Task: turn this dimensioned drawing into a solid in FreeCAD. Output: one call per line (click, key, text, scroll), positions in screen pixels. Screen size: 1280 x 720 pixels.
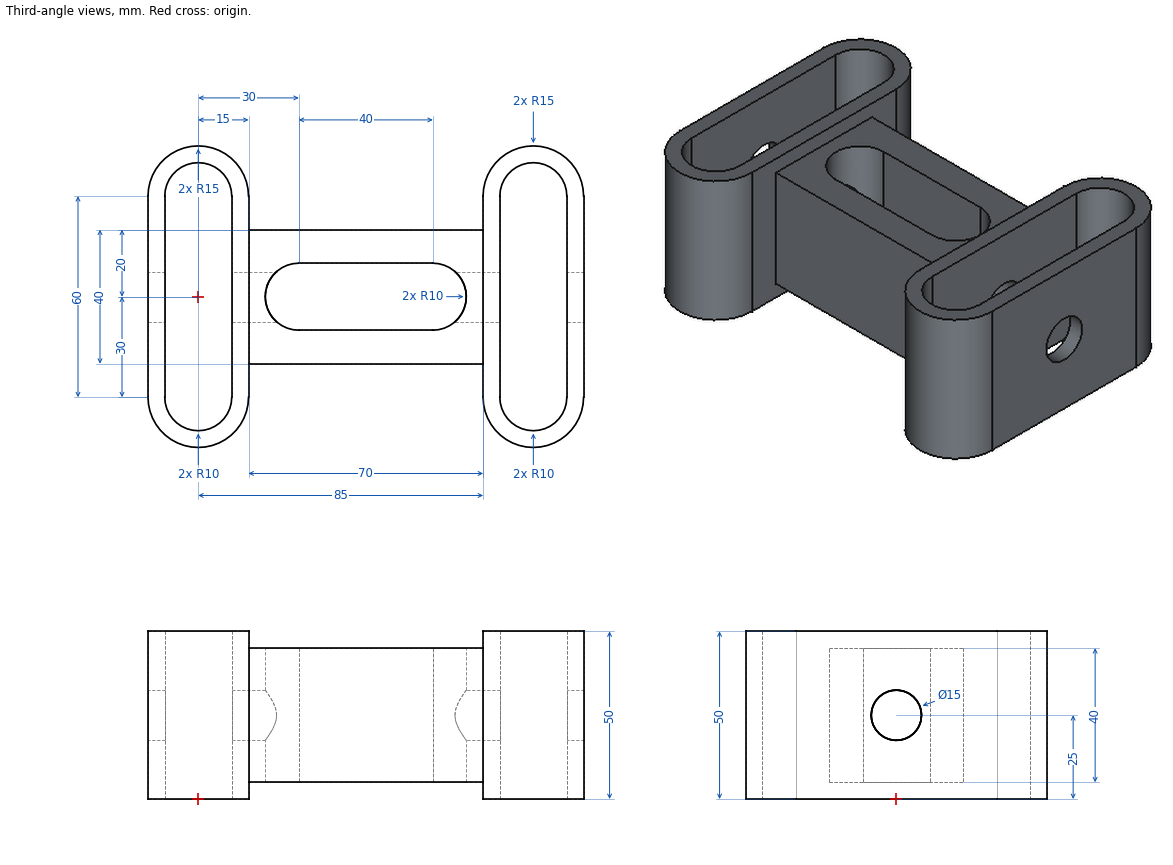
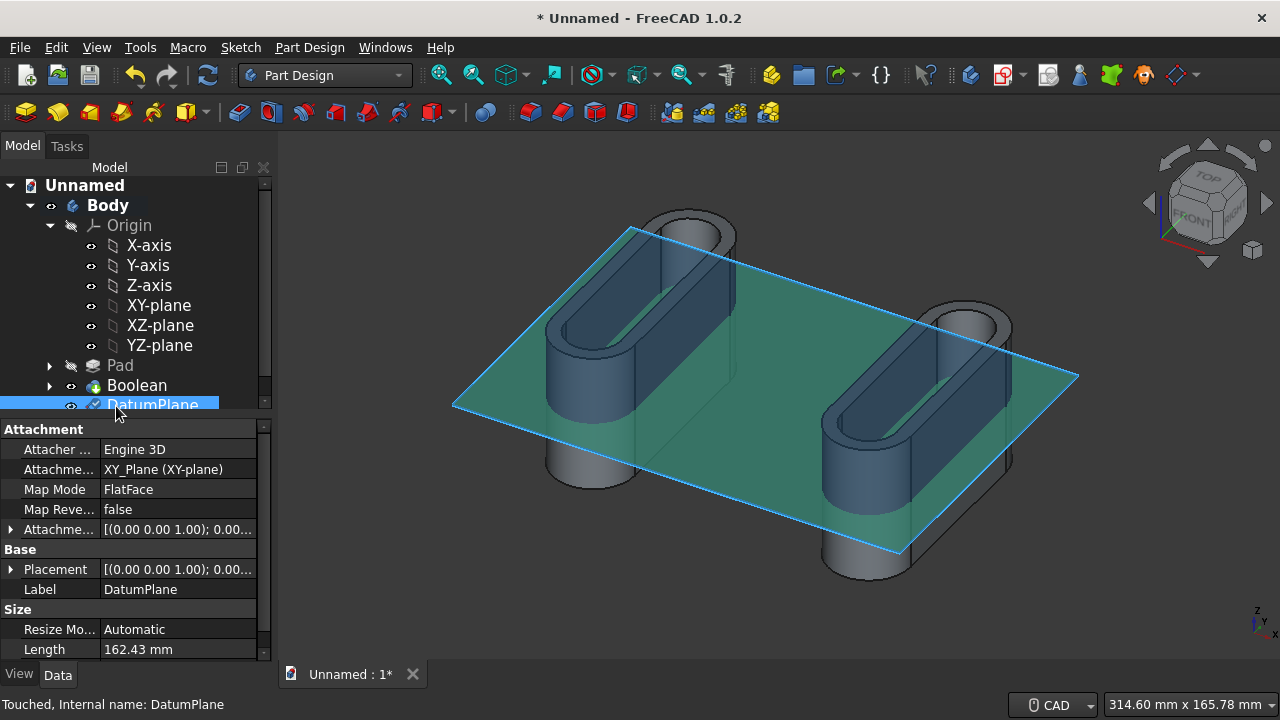
click(1004, 76)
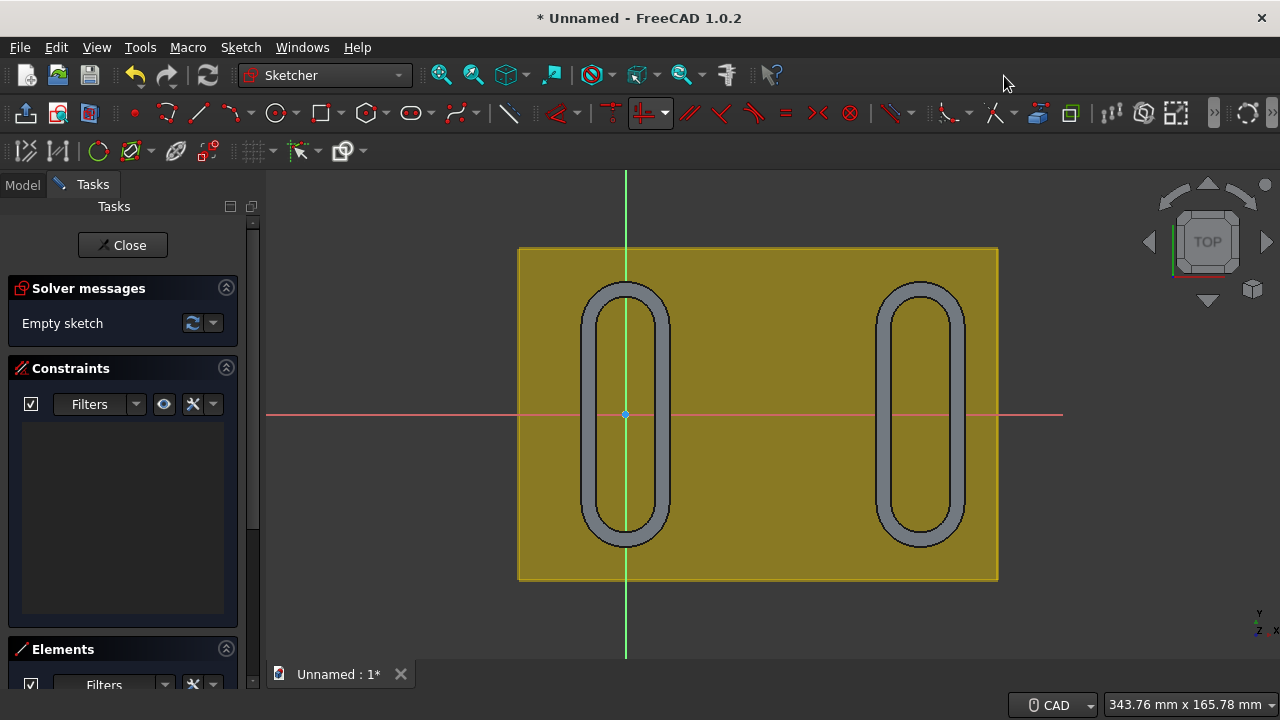
click(90, 114)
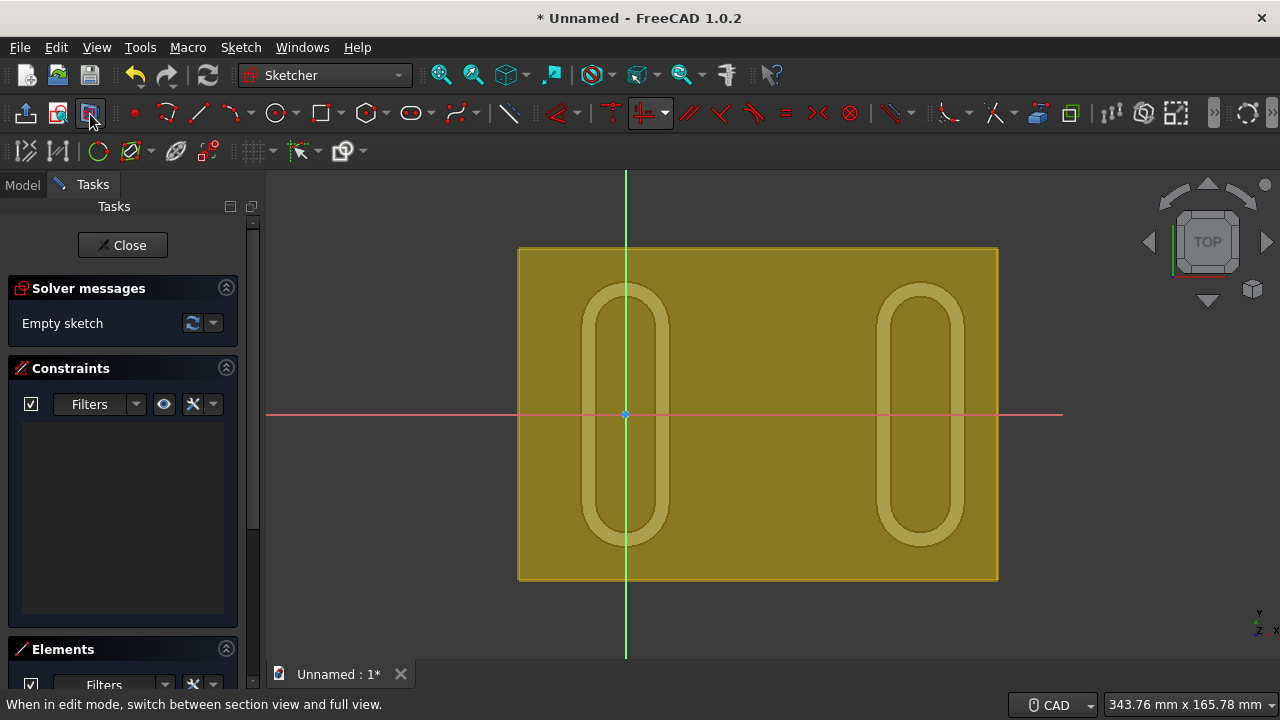
scroll(789, 414, up, 4)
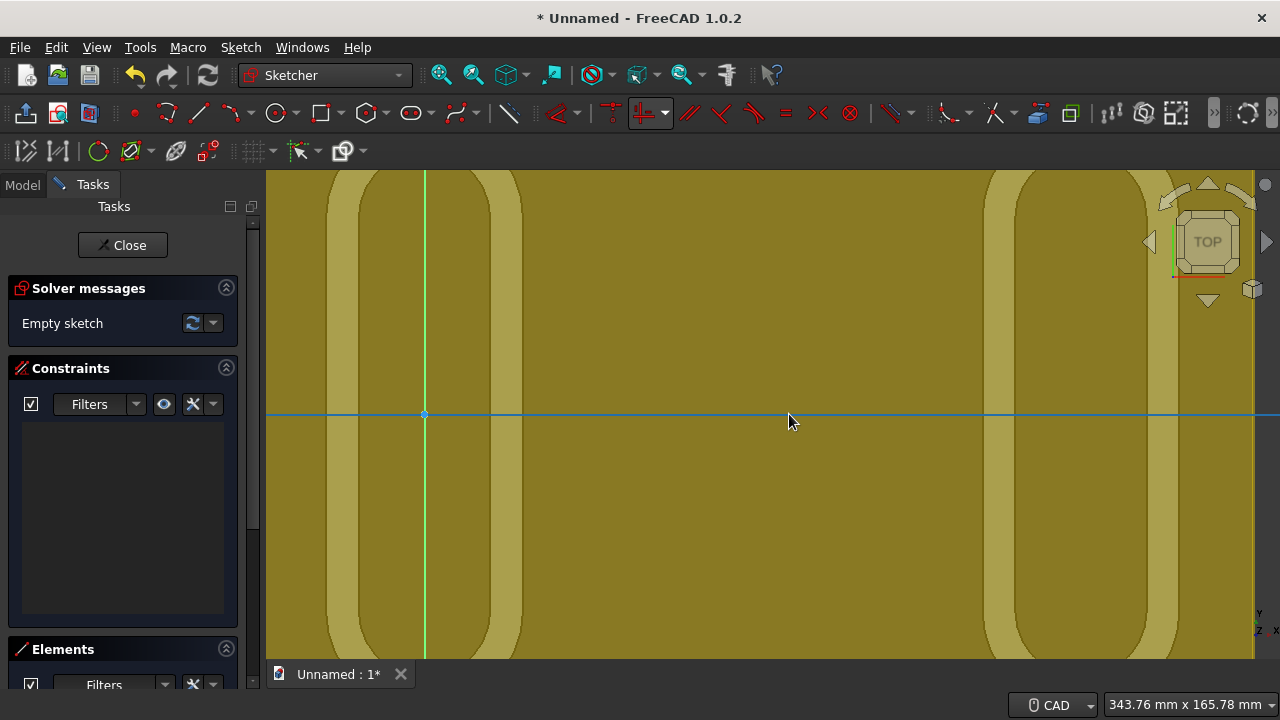
click(322, 114)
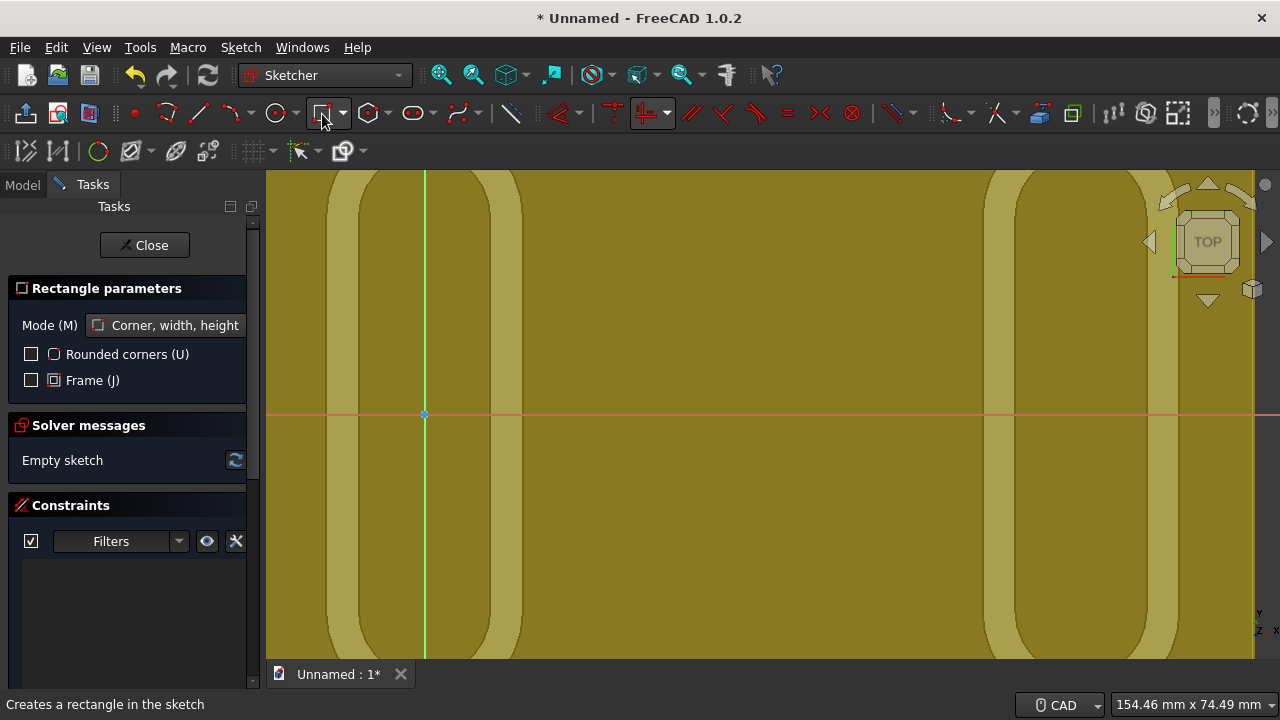
click(523, 283)
click(983, 546)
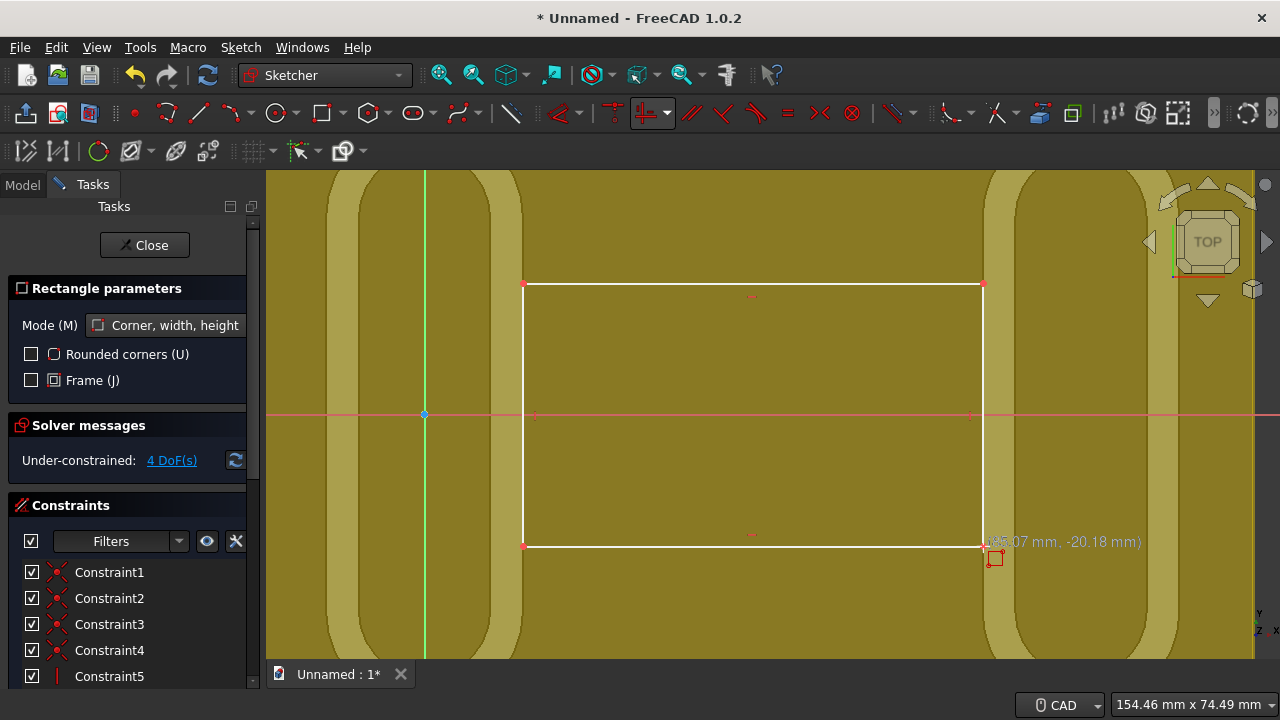
click(414, 114)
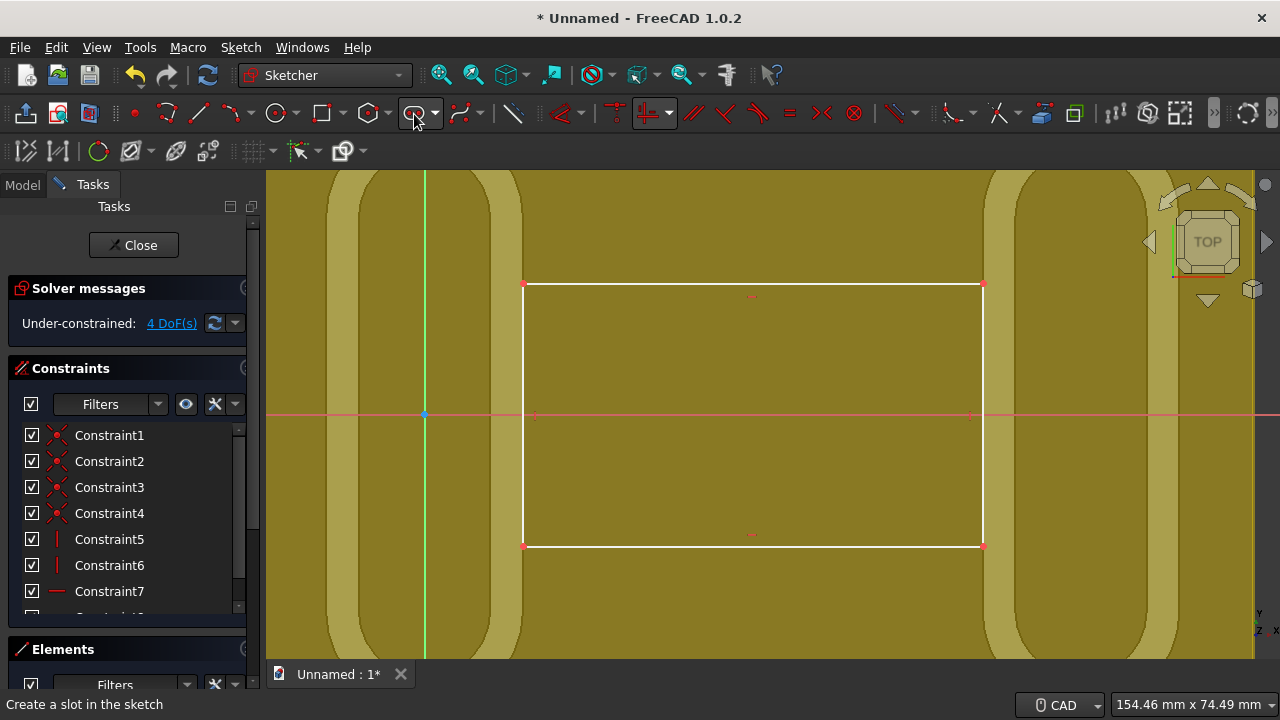
click(621, 414)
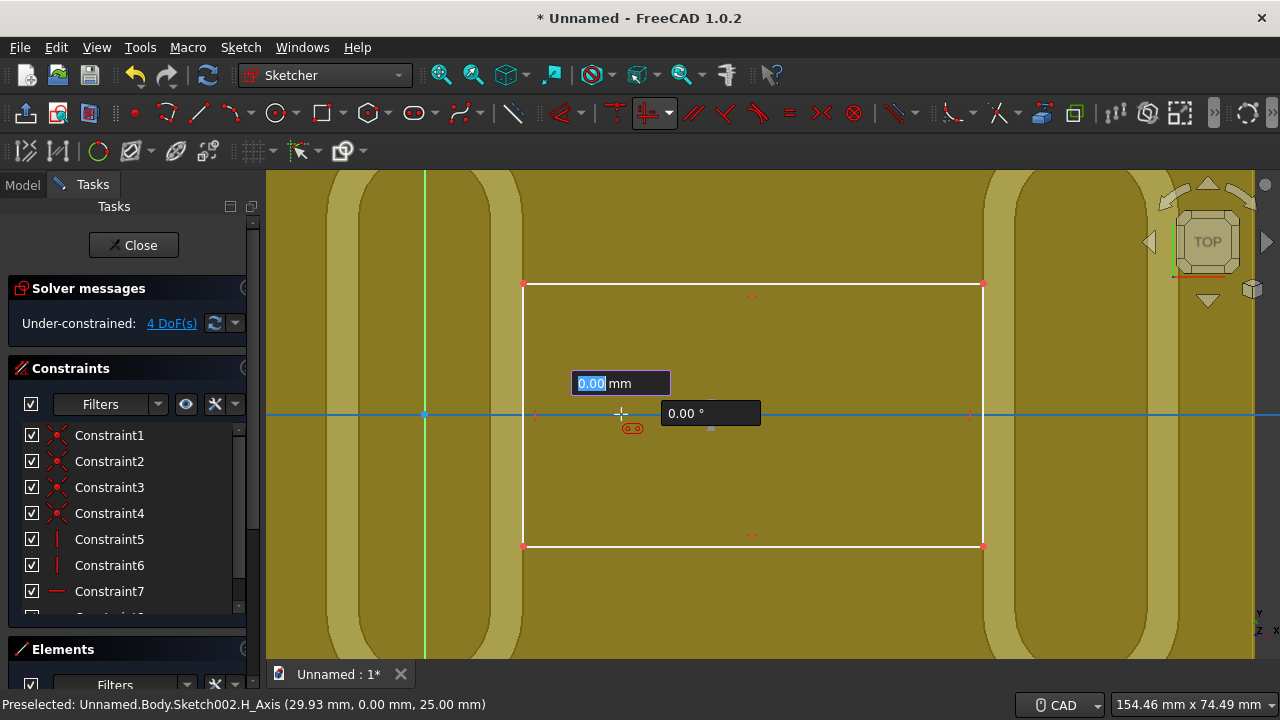
click(884, 406)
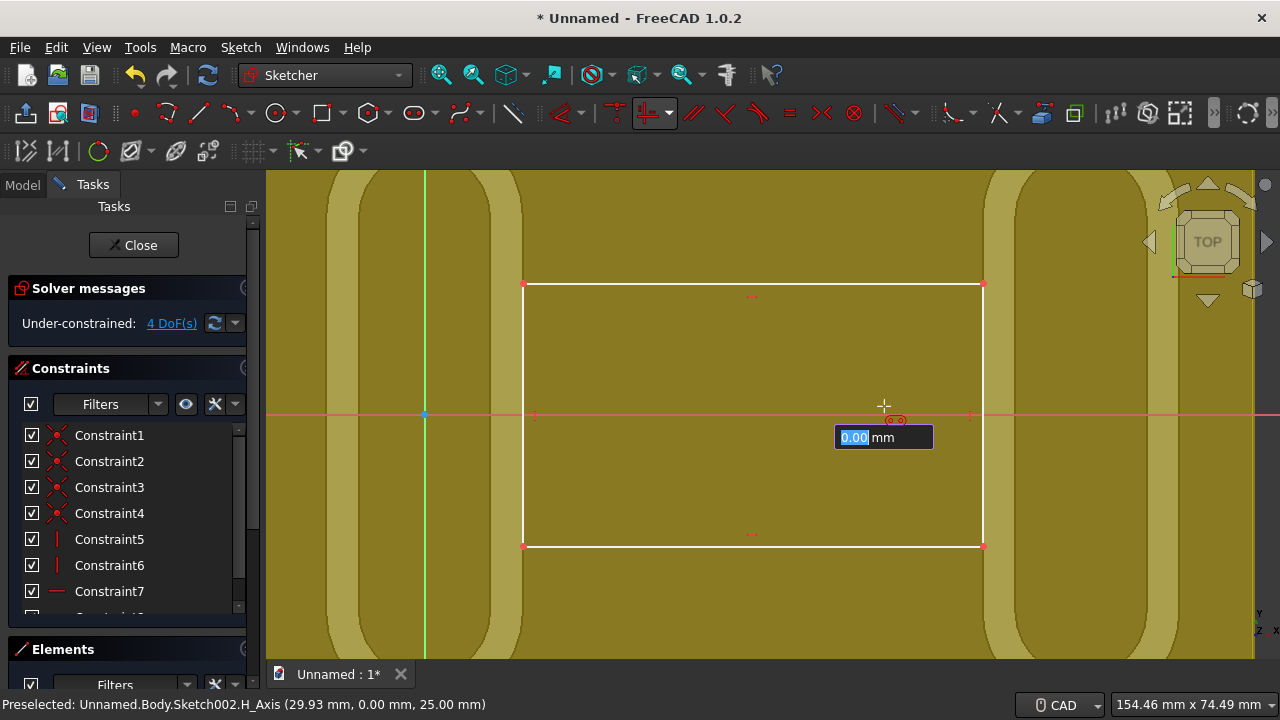
click(753, 480)
key(Escape)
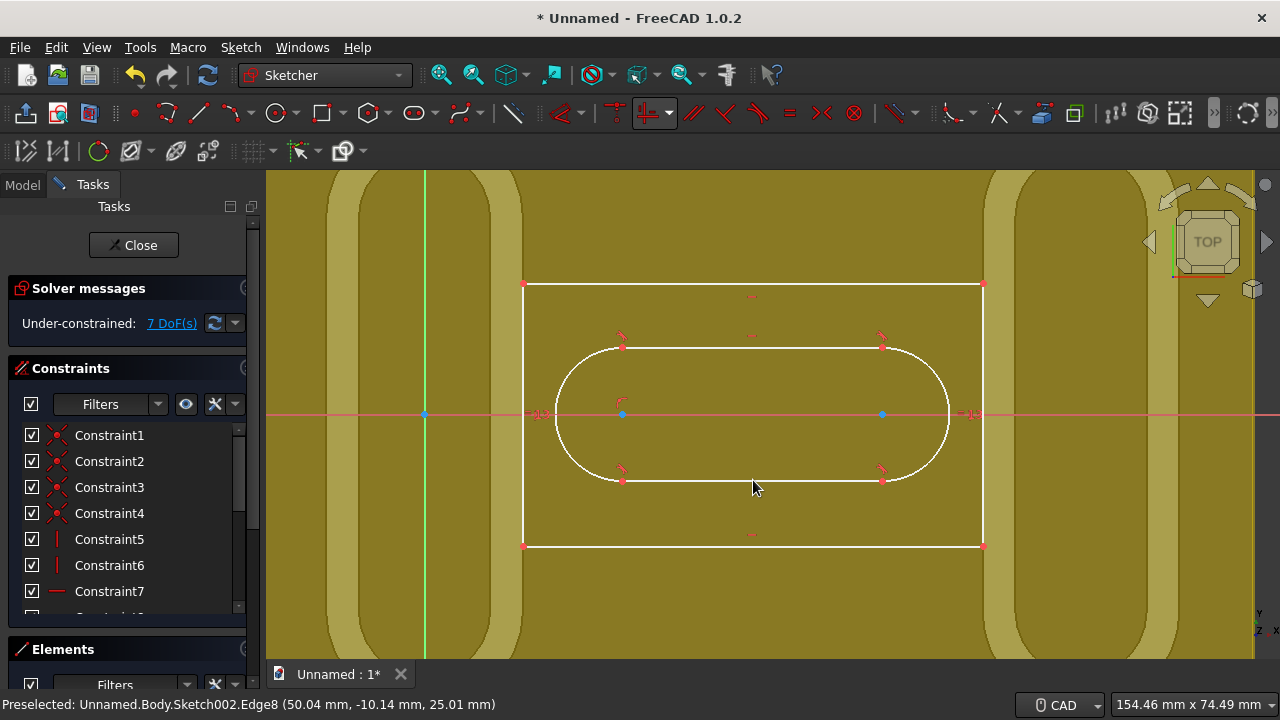
click(560, 114)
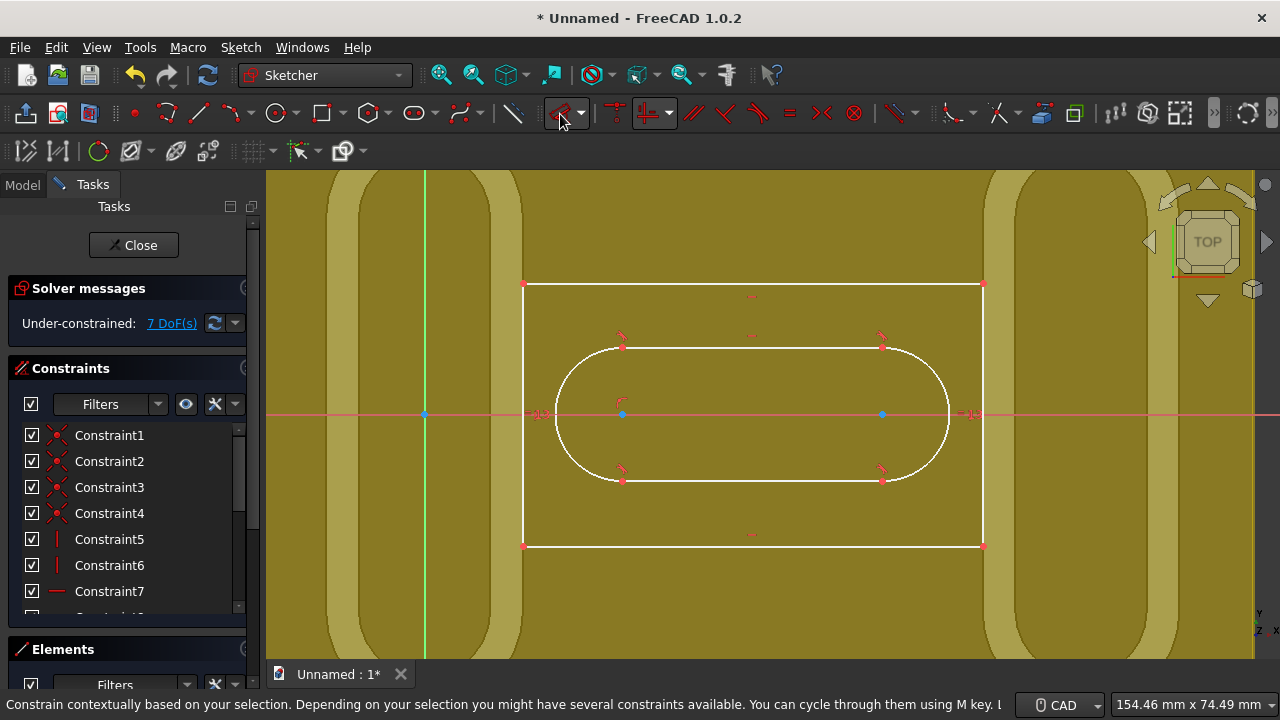
click(568, 375)
click(542, 356)